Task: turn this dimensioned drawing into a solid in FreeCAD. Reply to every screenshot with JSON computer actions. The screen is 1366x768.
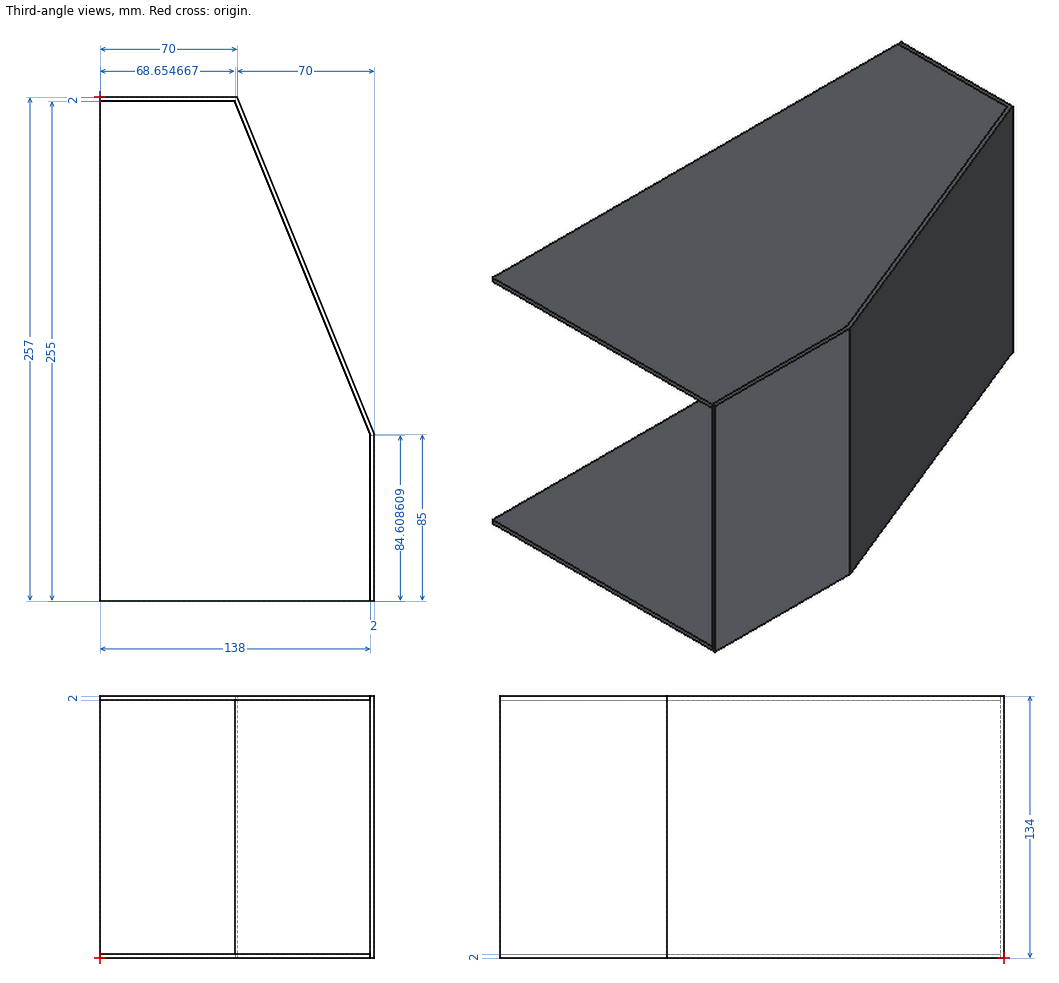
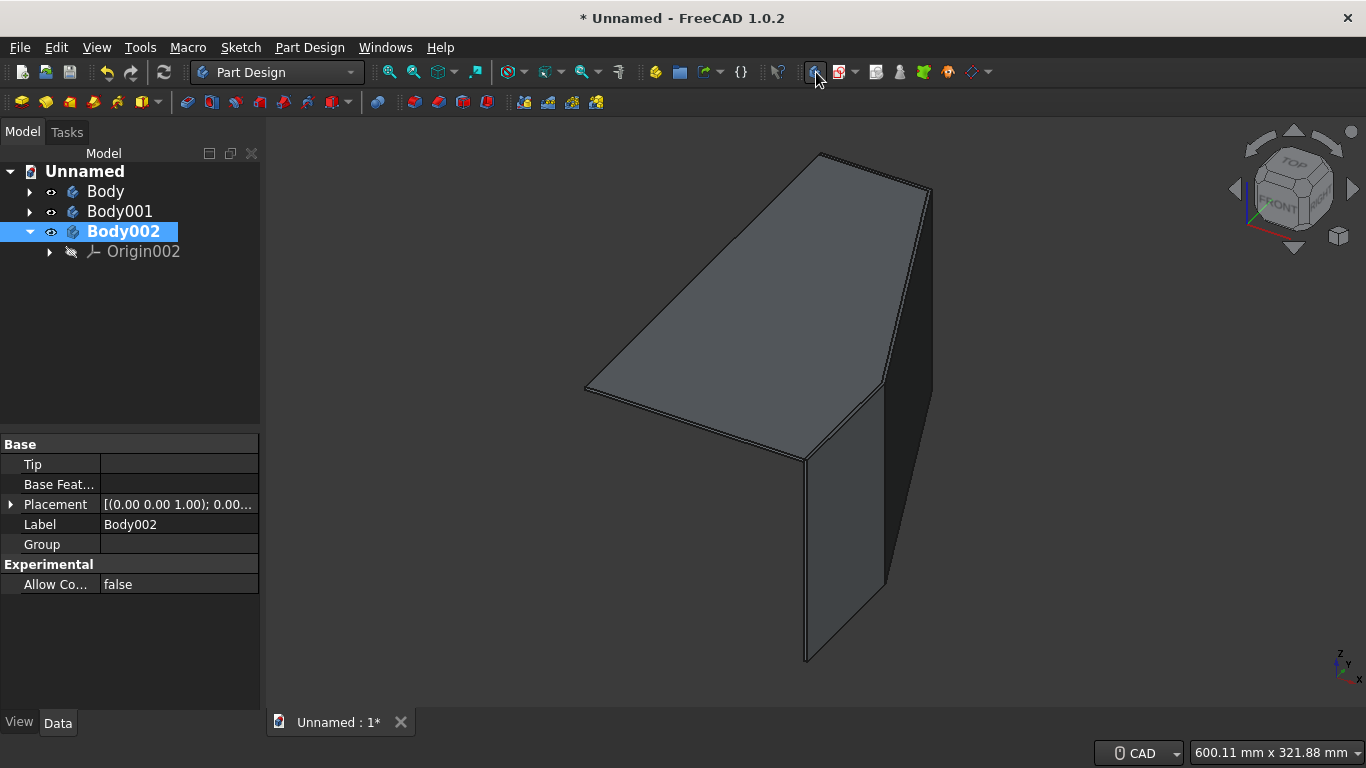
{"action": "left_click", "coordinate": [306, 667]}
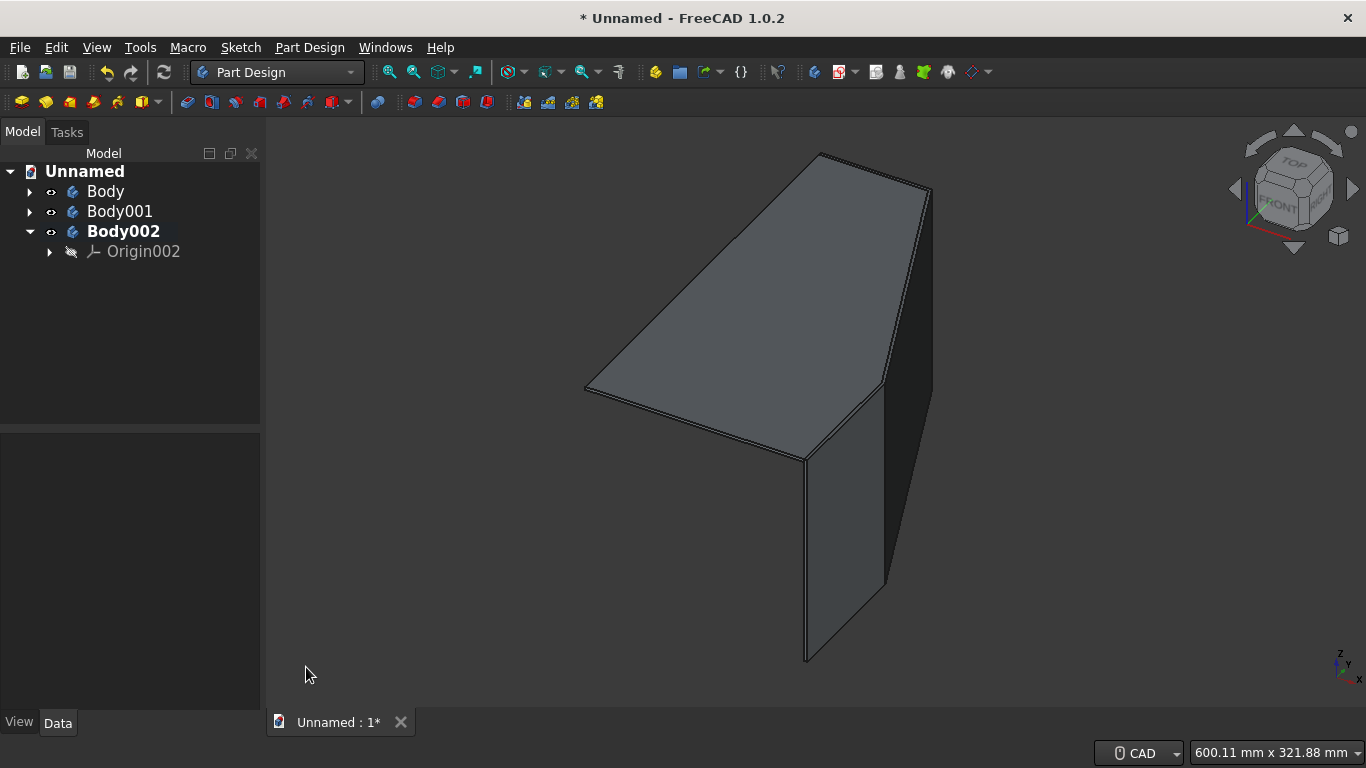
{"action": "left_click", "coordinate": [840, 72]}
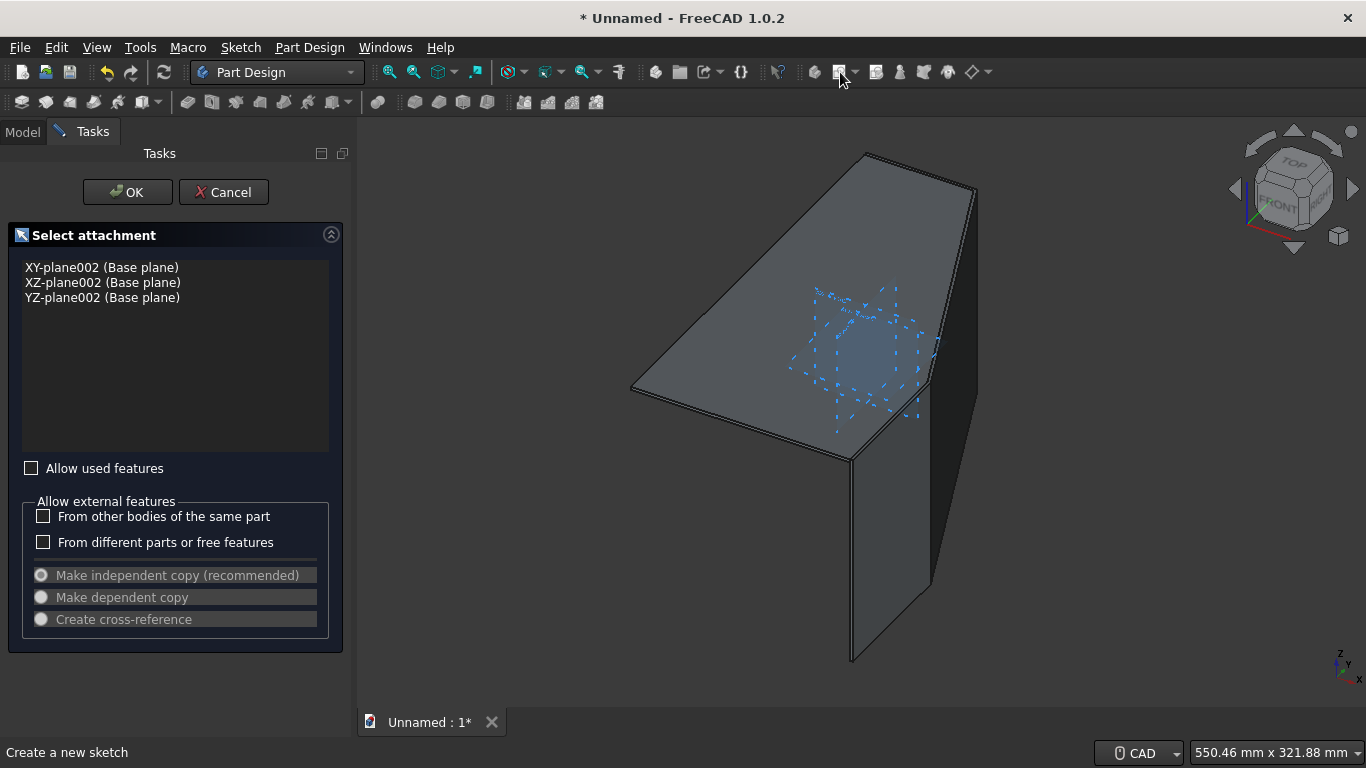
{"action": "left_click", "coordinate": [82, 268]}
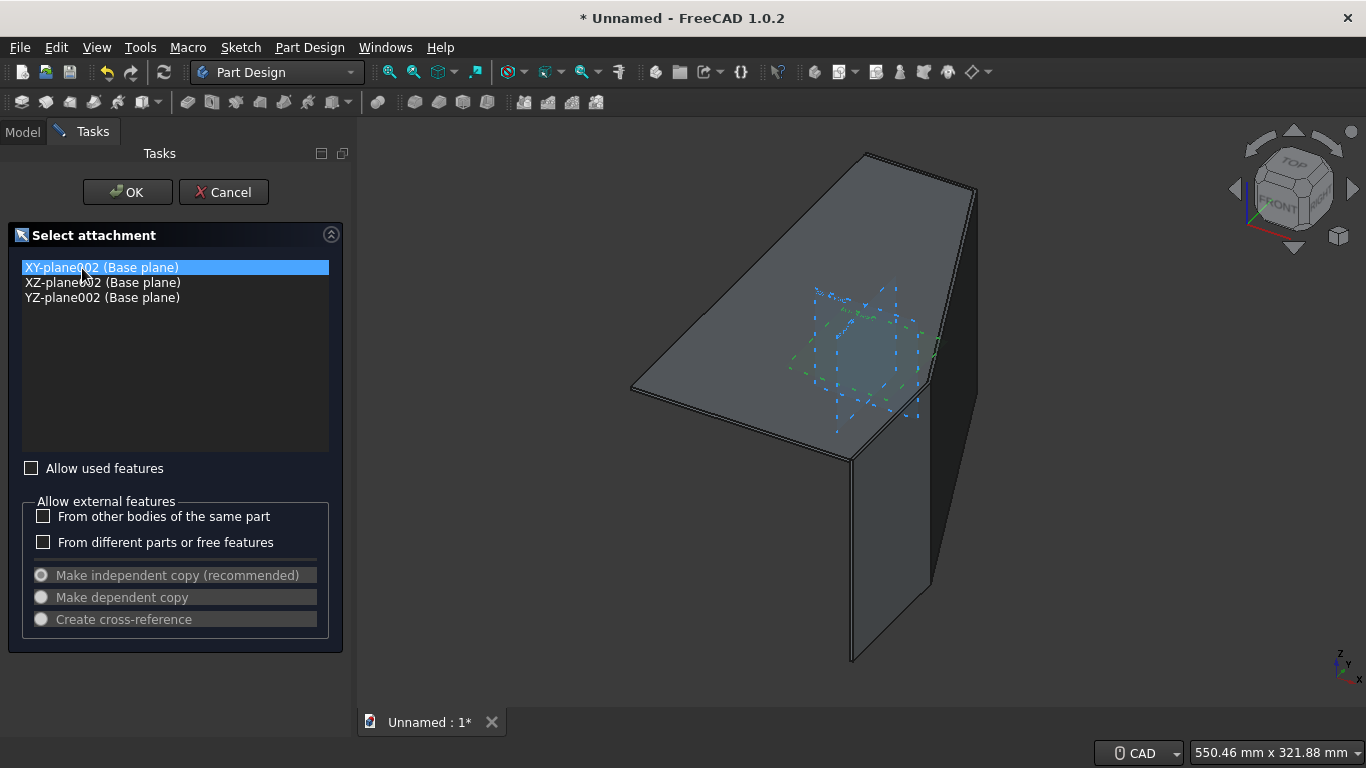
{"action": "left_click", "coordinate": [128, 192]}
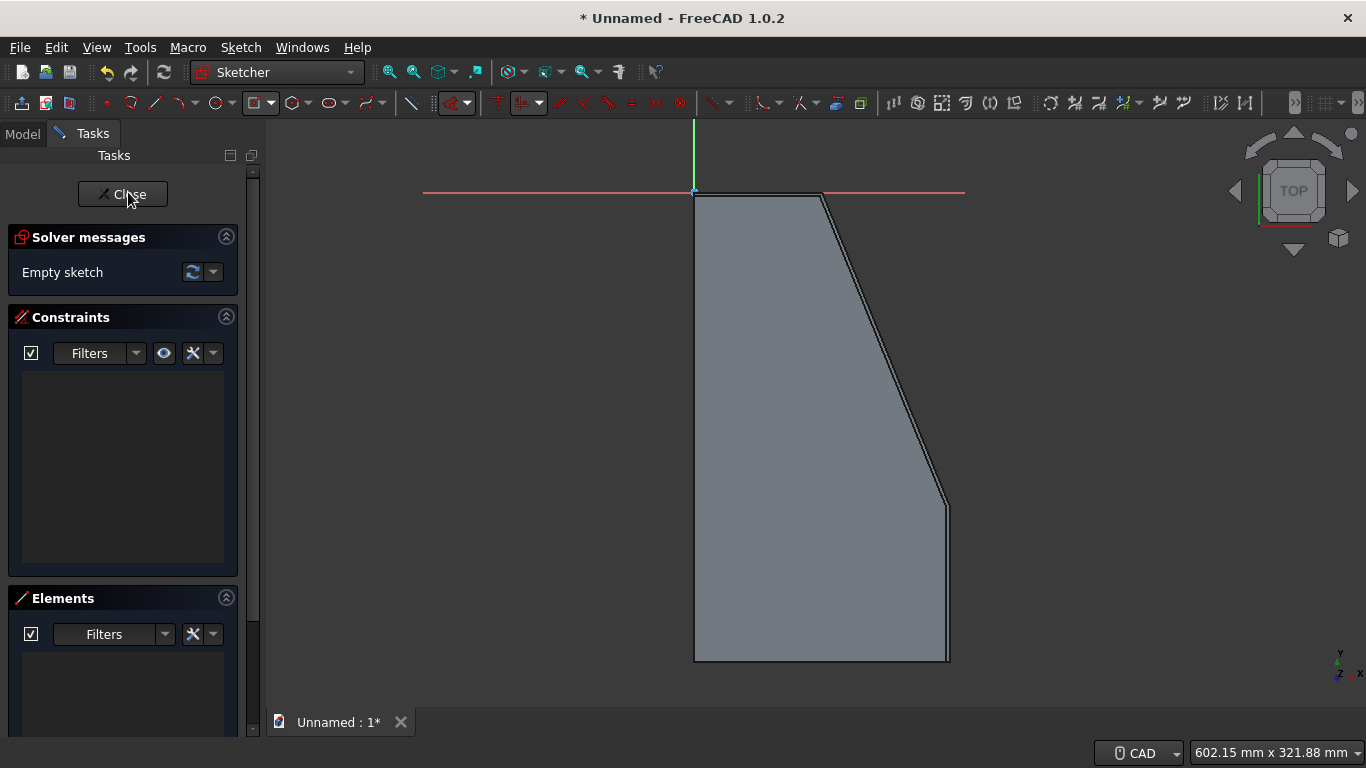
{"action": "scroll", "coordinate": [418, 348], "scroll_direction": "down", "scroll_amount": 1}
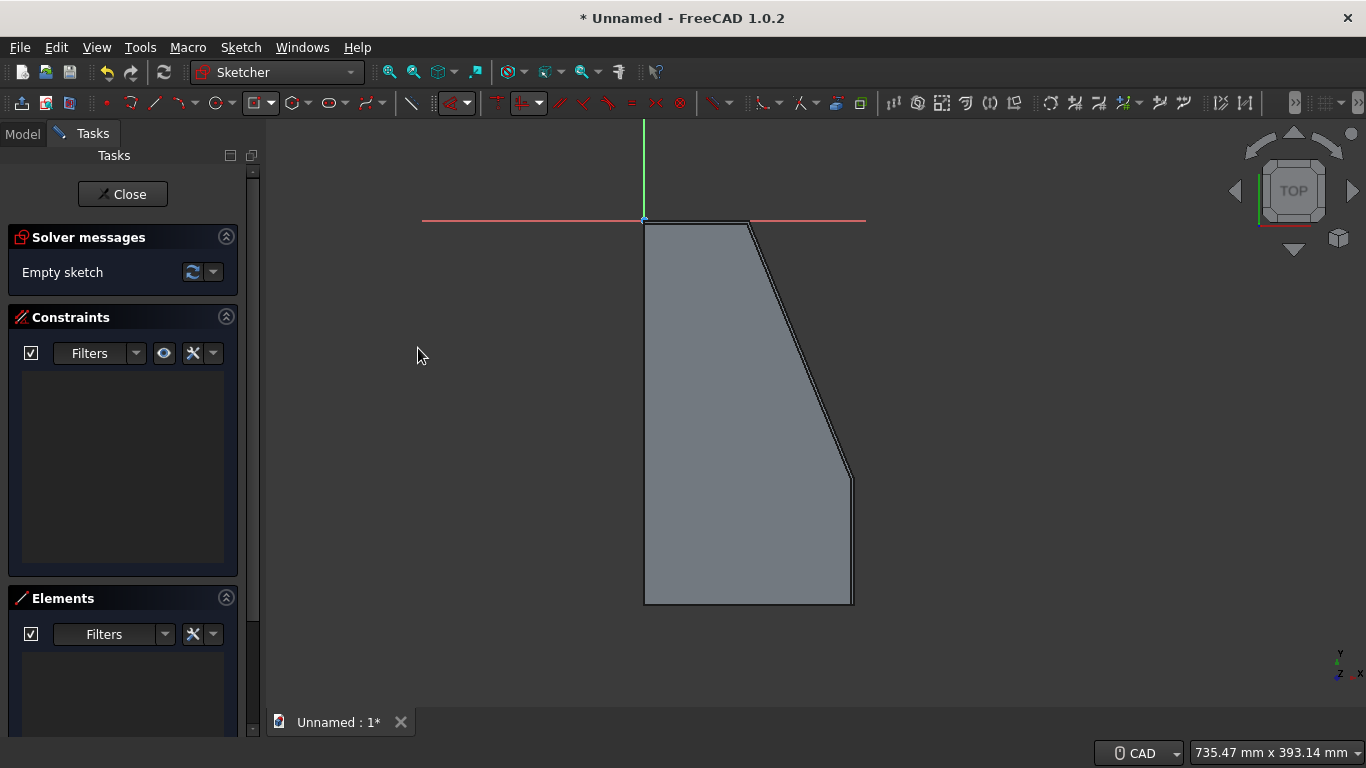
{"action": "key", "text": "g m"}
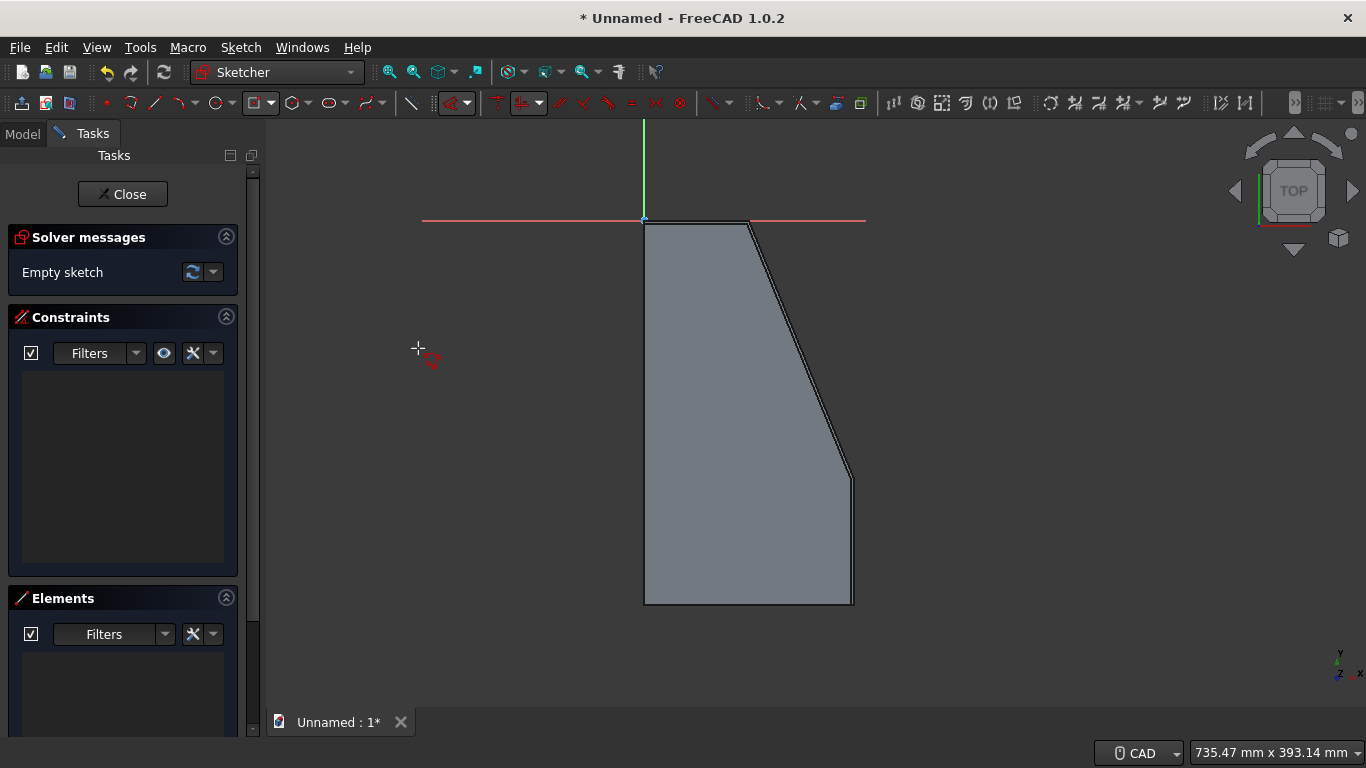
{"action": "scroll", "coordinate": [644, 224], "scroll_direction": "up", "scroll_amount": 9}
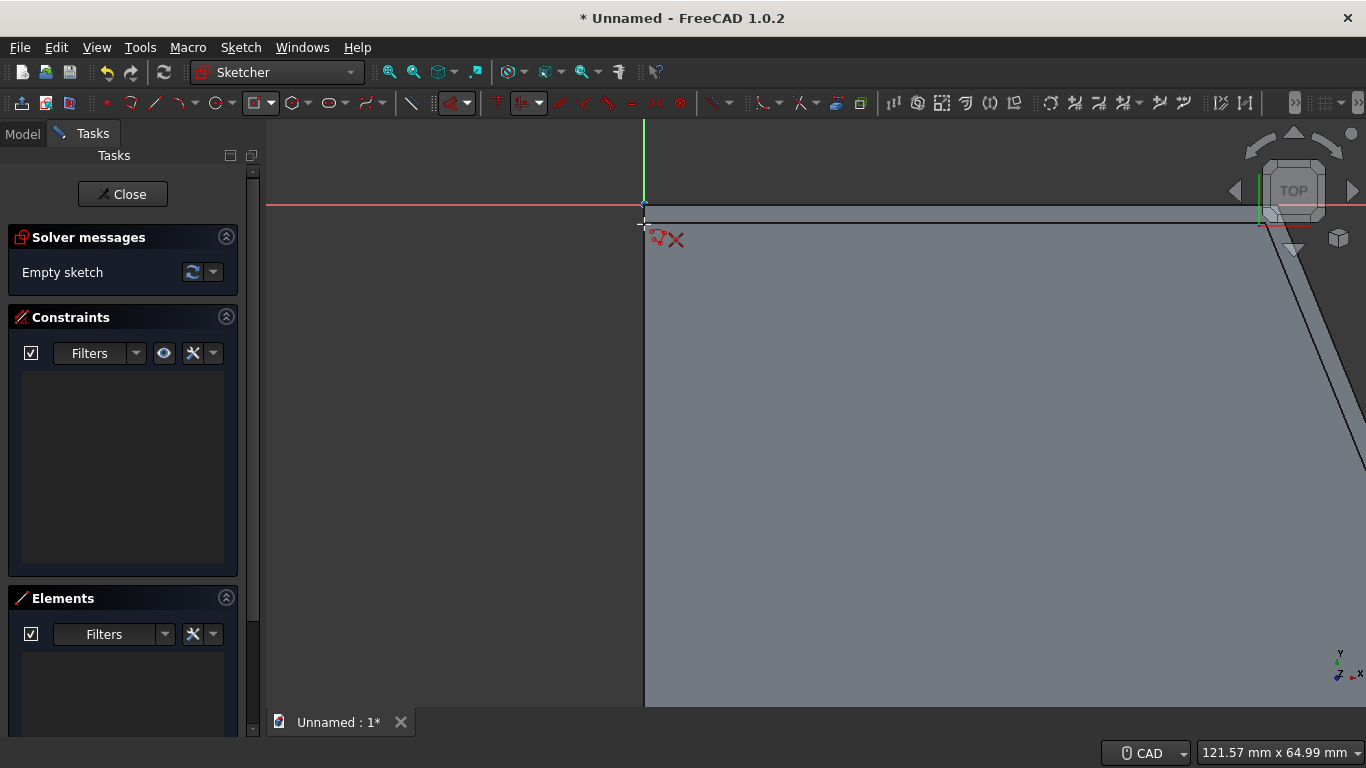
{"action": "left_click", "coordinate": [644, 223]}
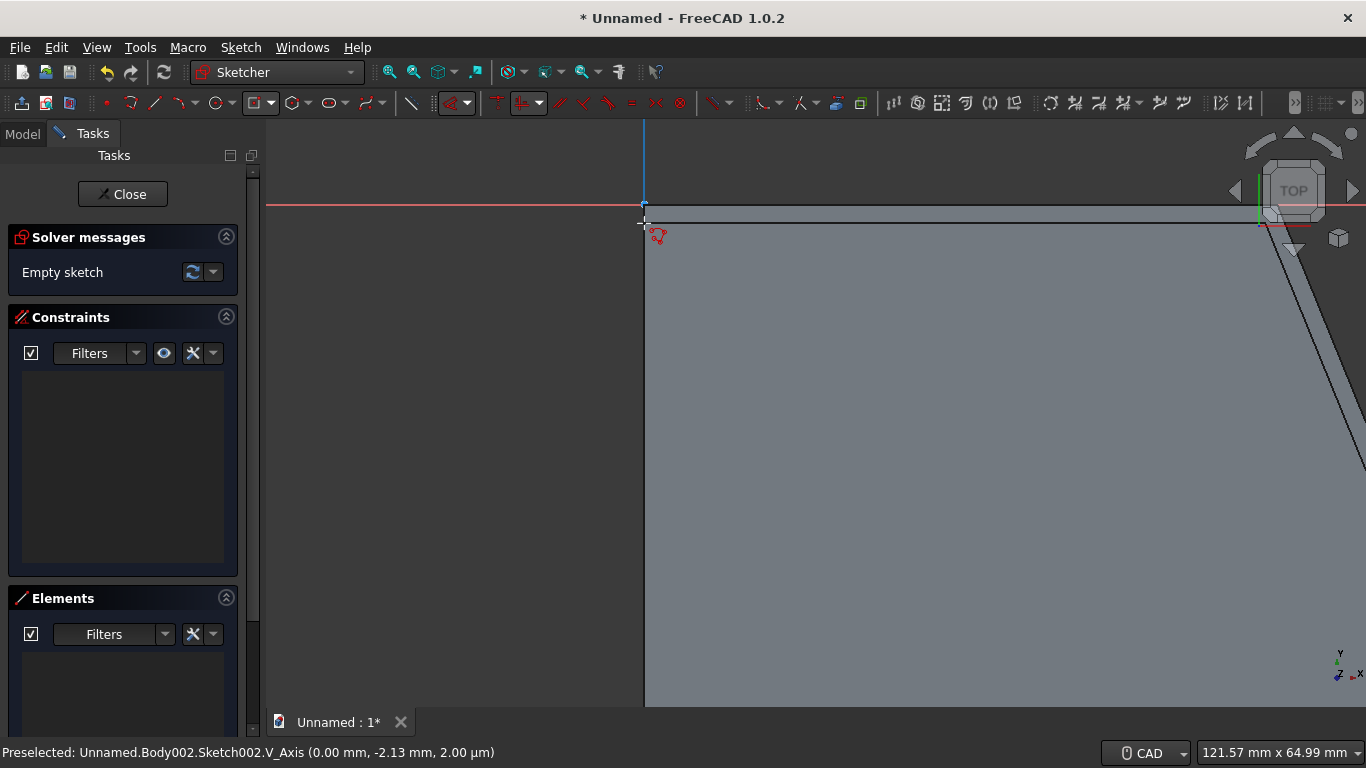
{"action": "scroll", "coordinate": [644, 224], "scroll_direction": "down", "scroll_amount": 9}